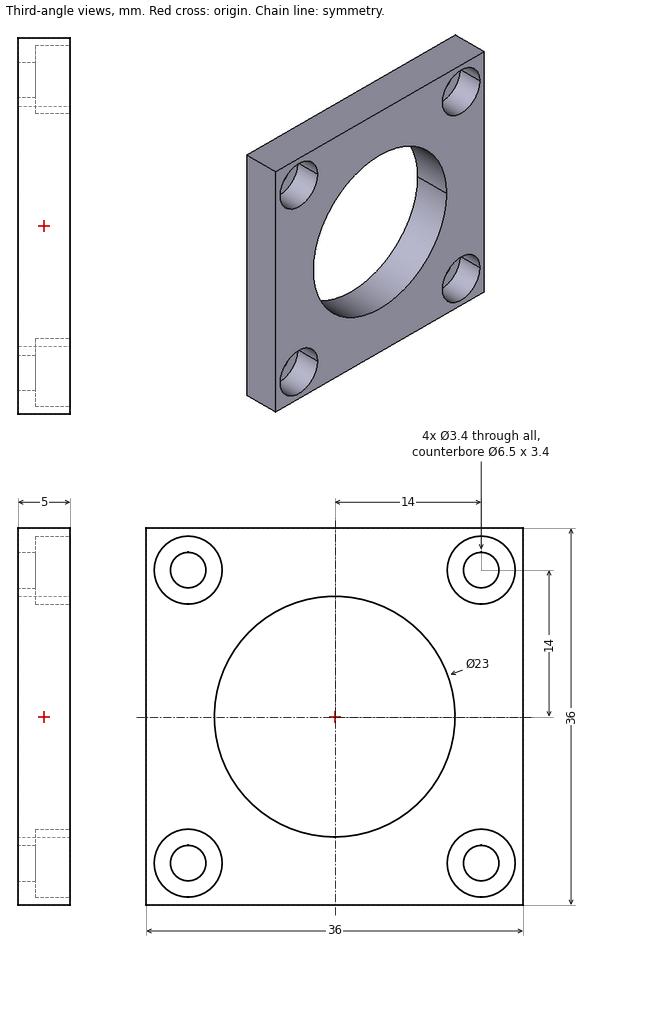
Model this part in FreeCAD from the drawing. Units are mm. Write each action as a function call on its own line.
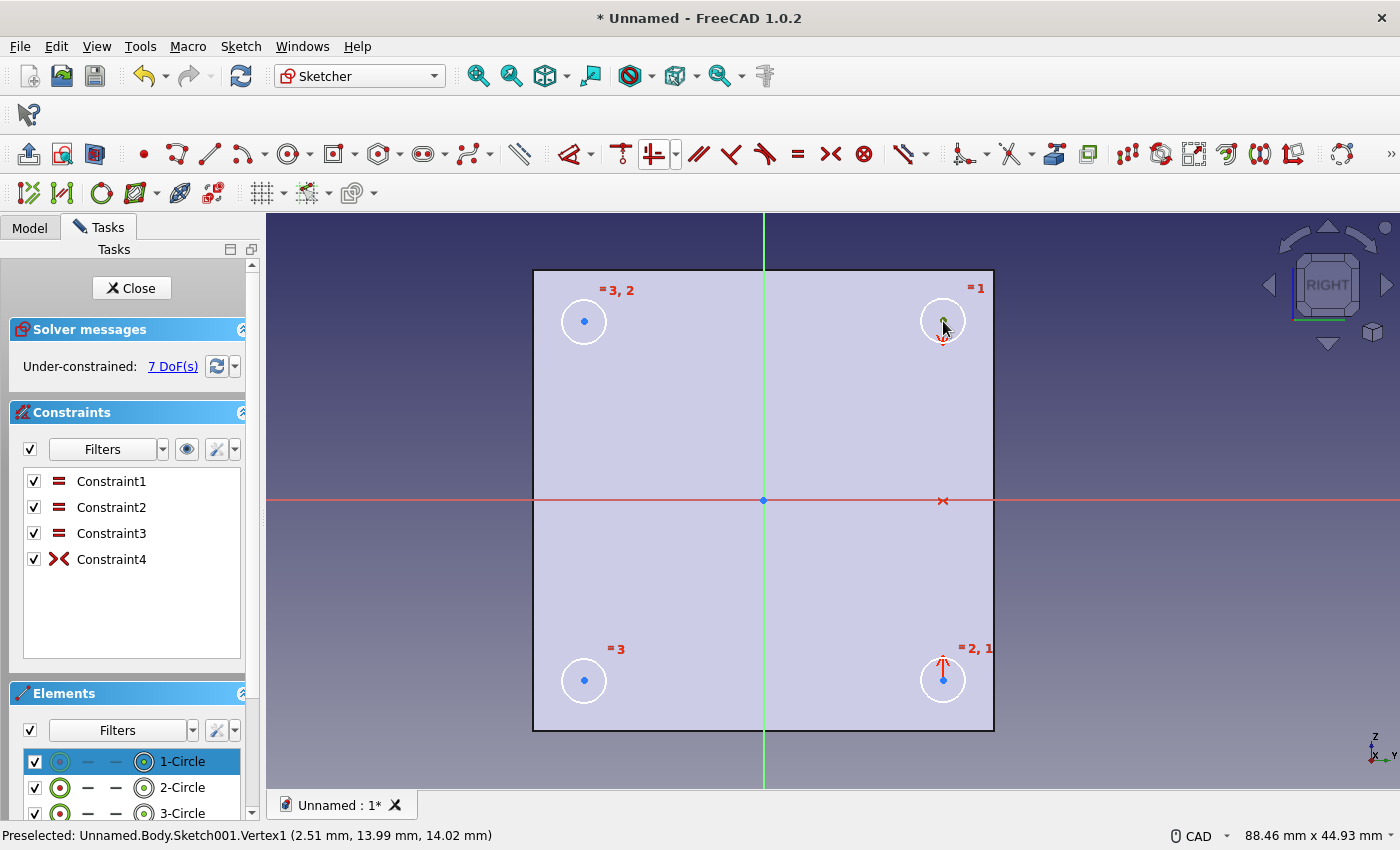
click(584, 322)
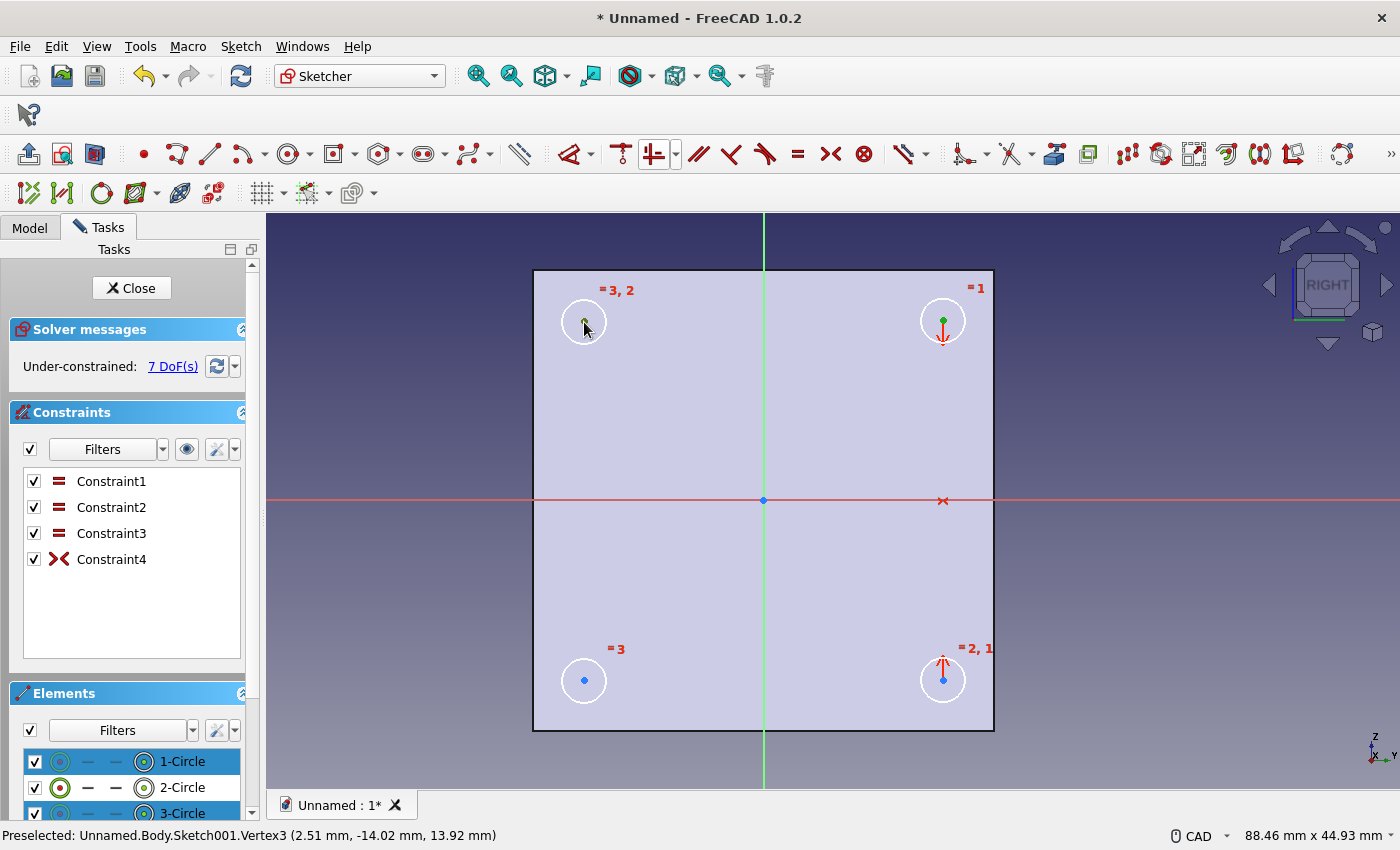
click(764, 724)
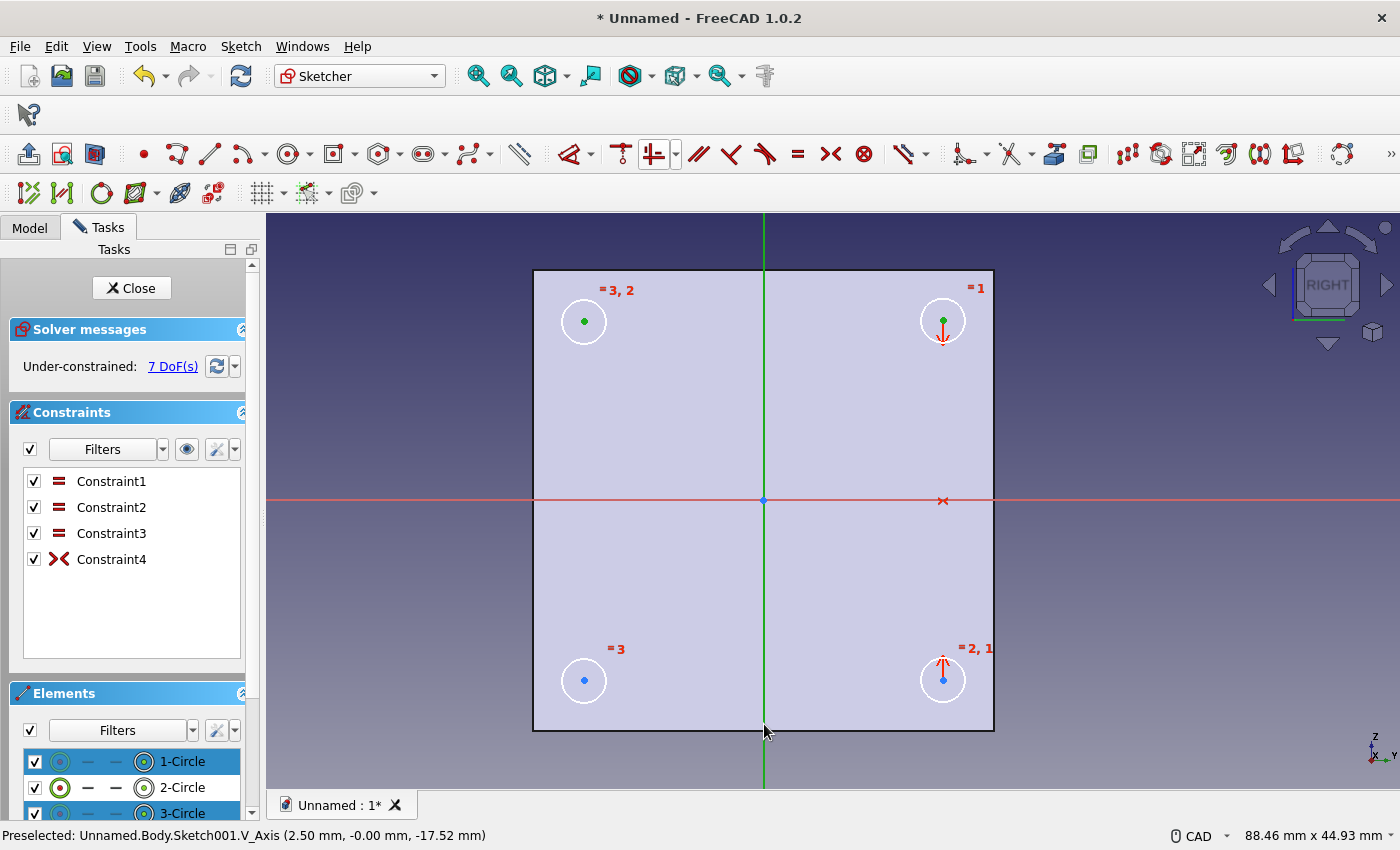
click(831, 154)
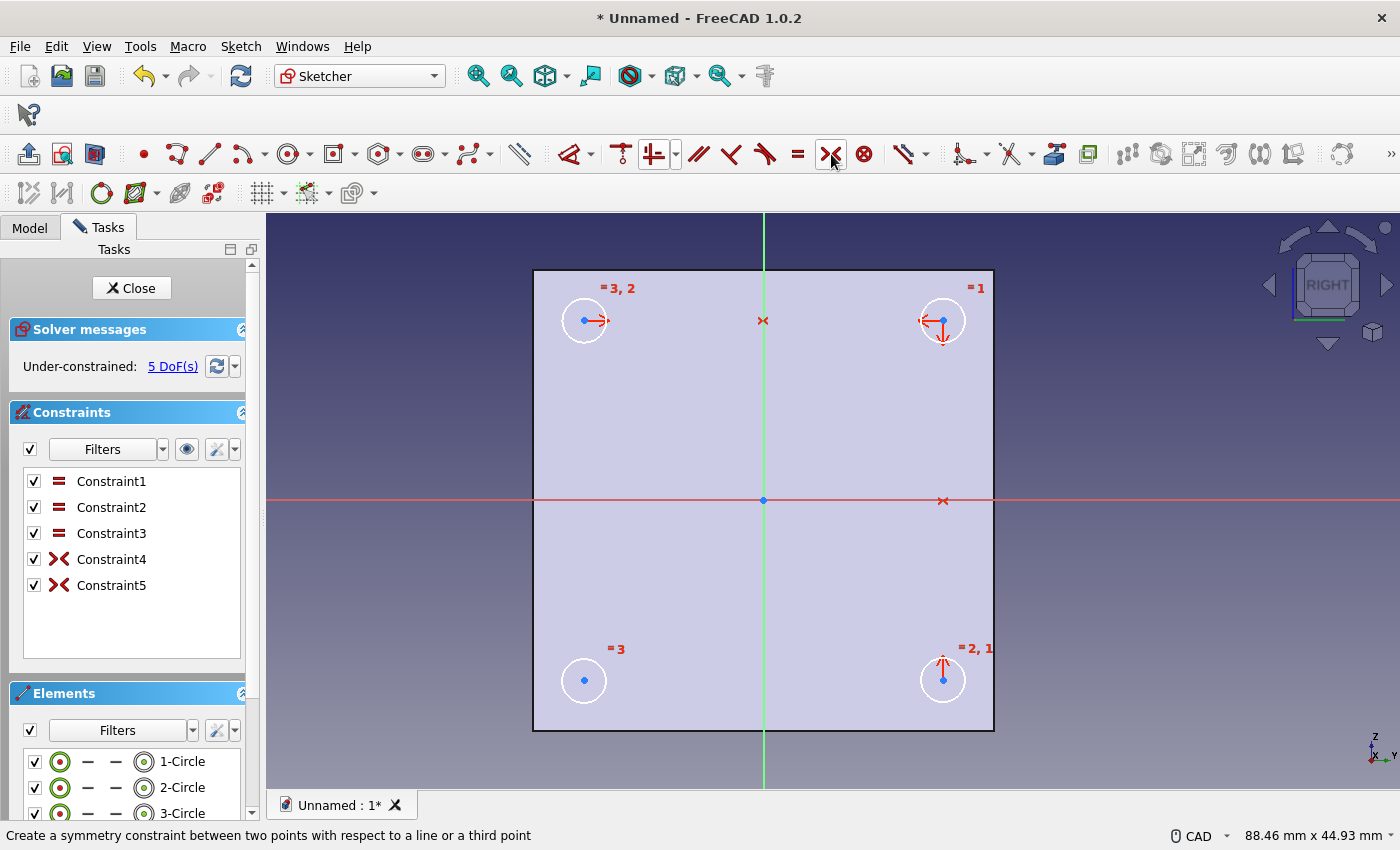
click(943, 680)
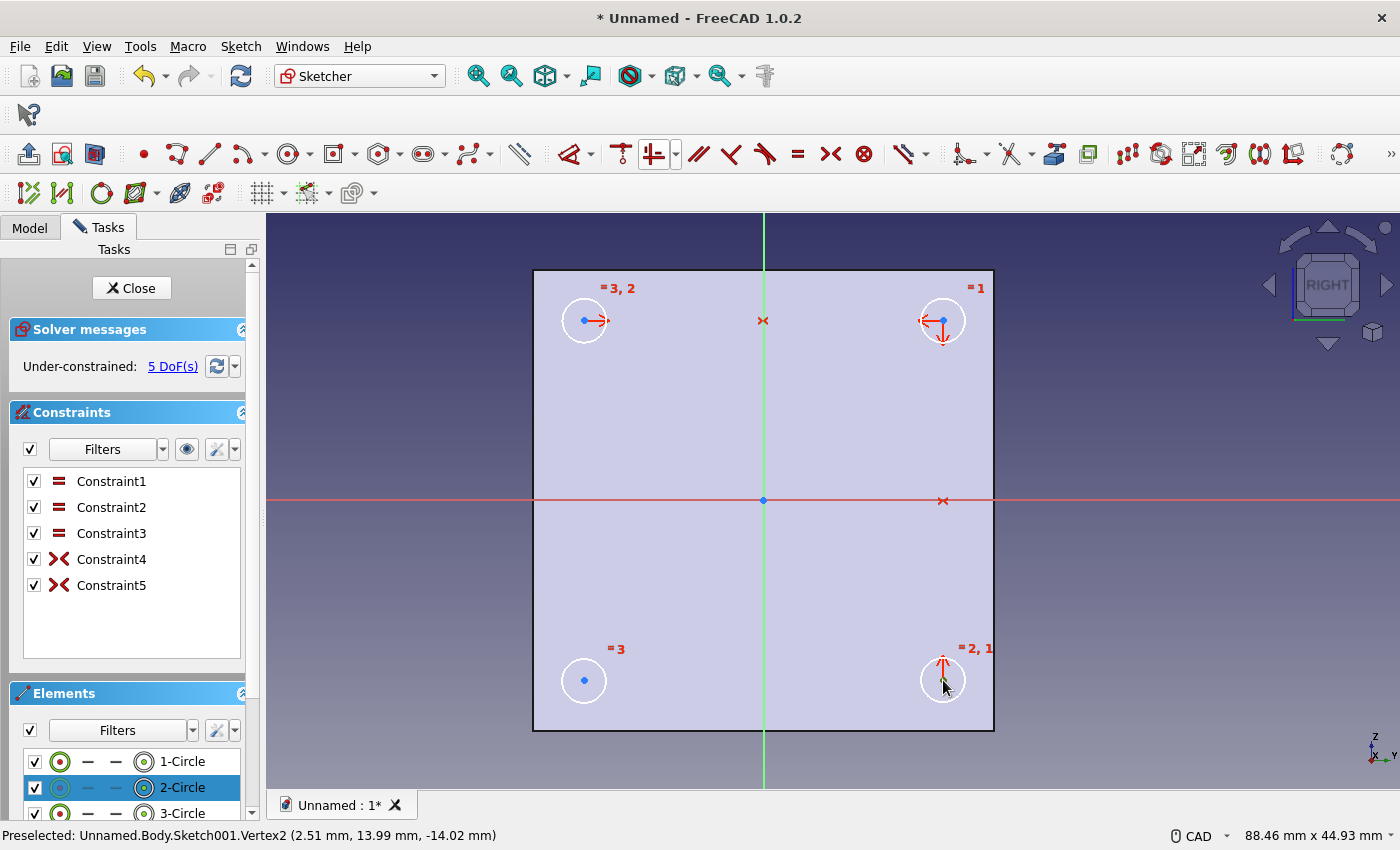
click(584, 681)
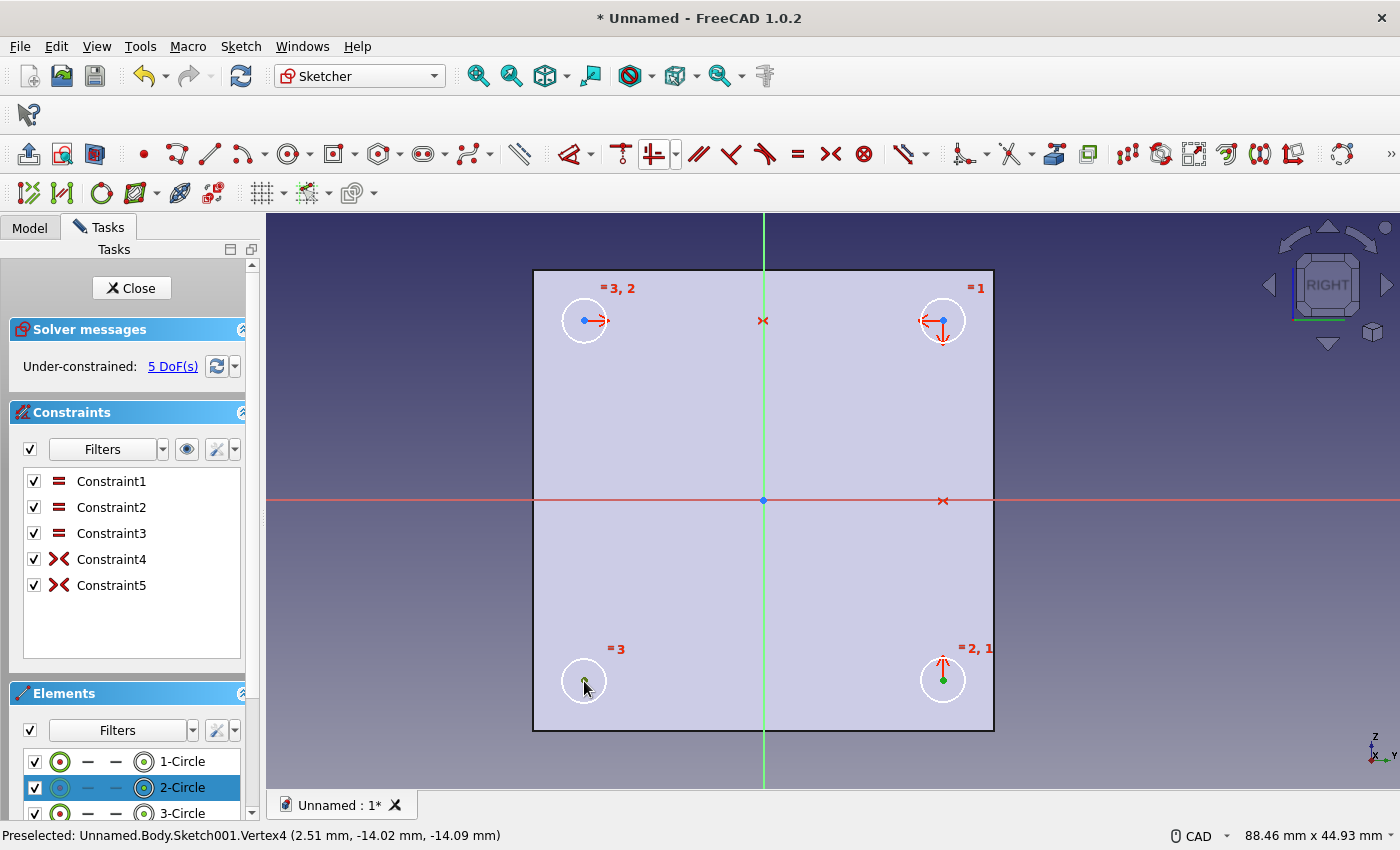
click(764, 724)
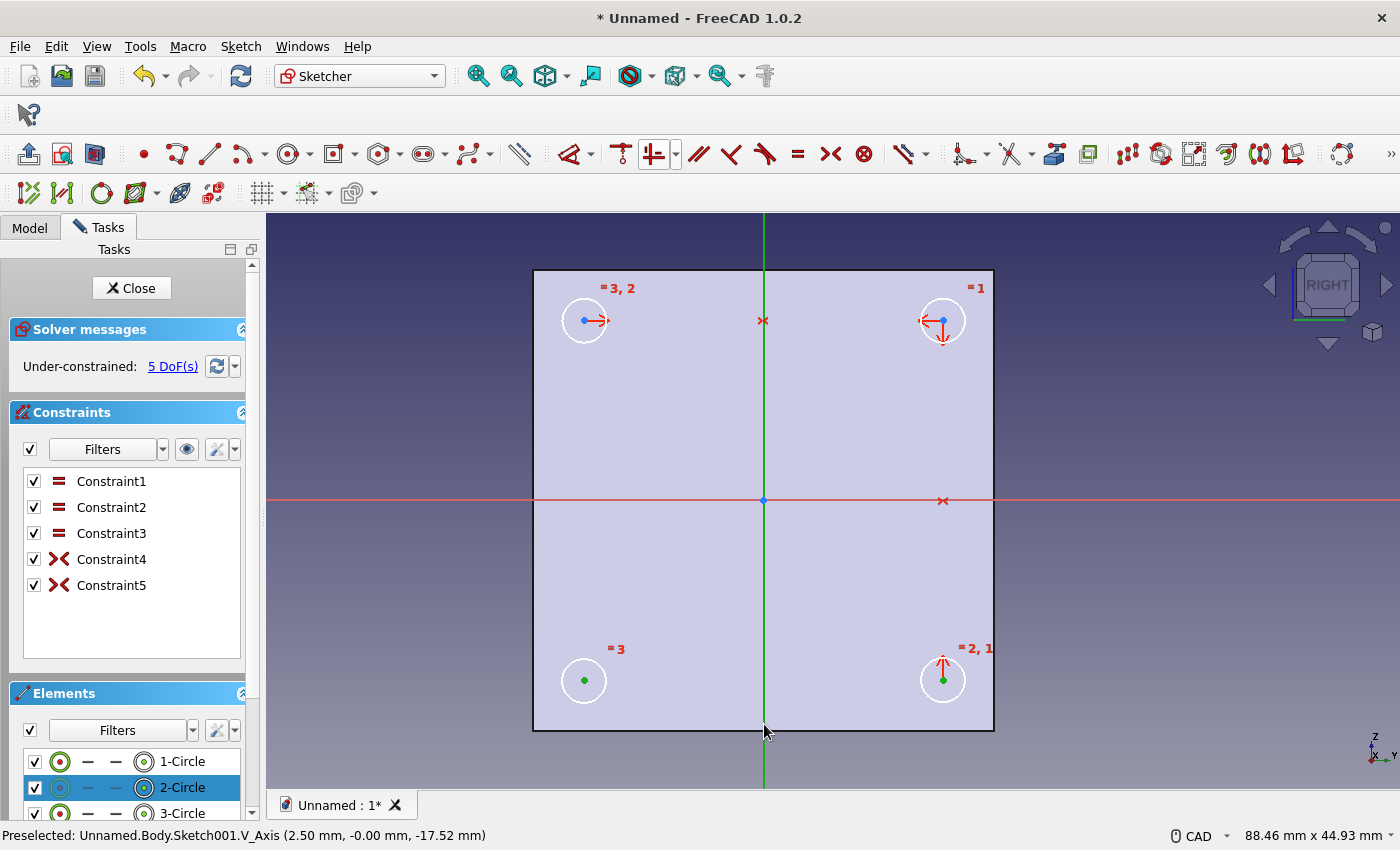
click(831, 154)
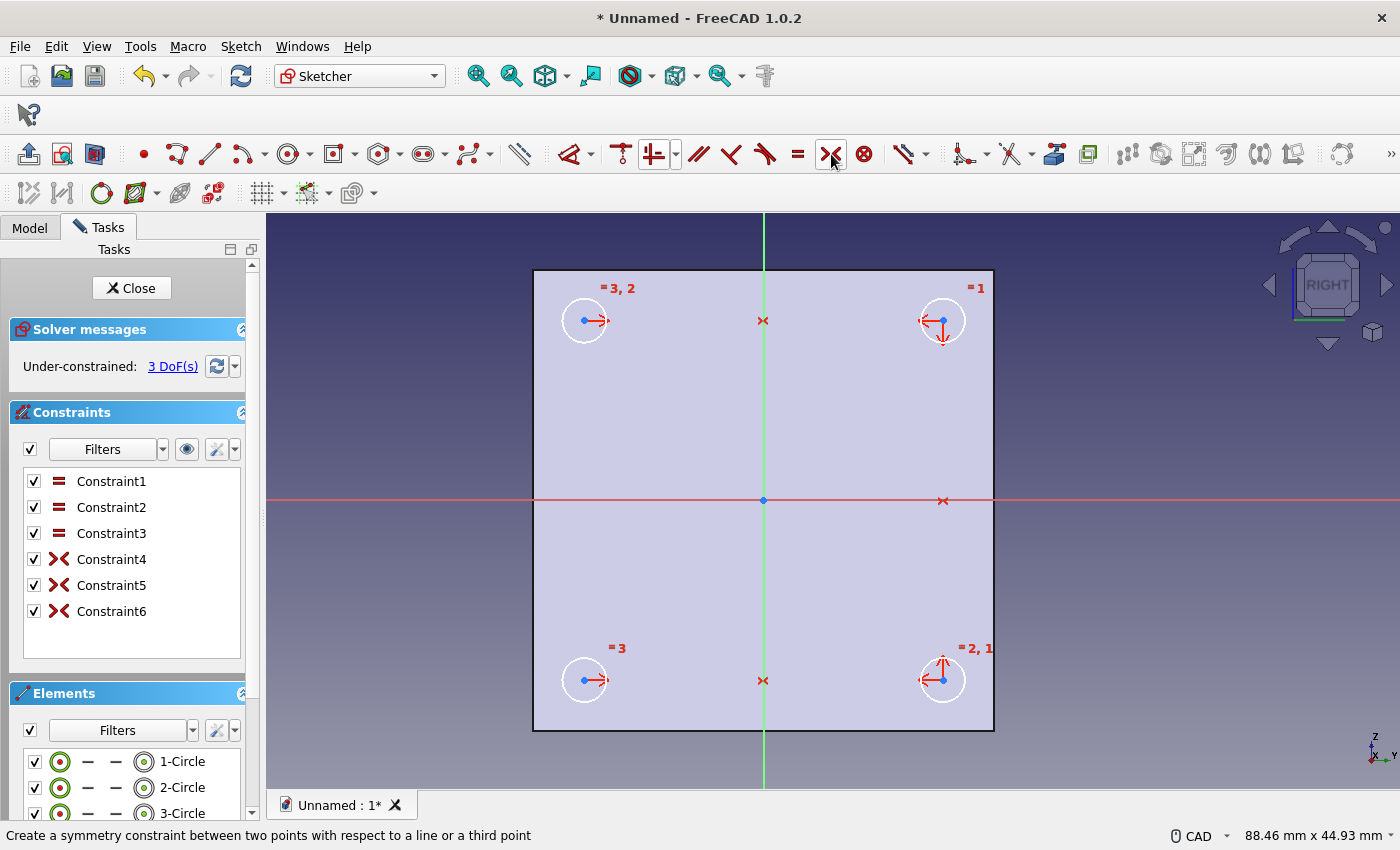
click(958, 305)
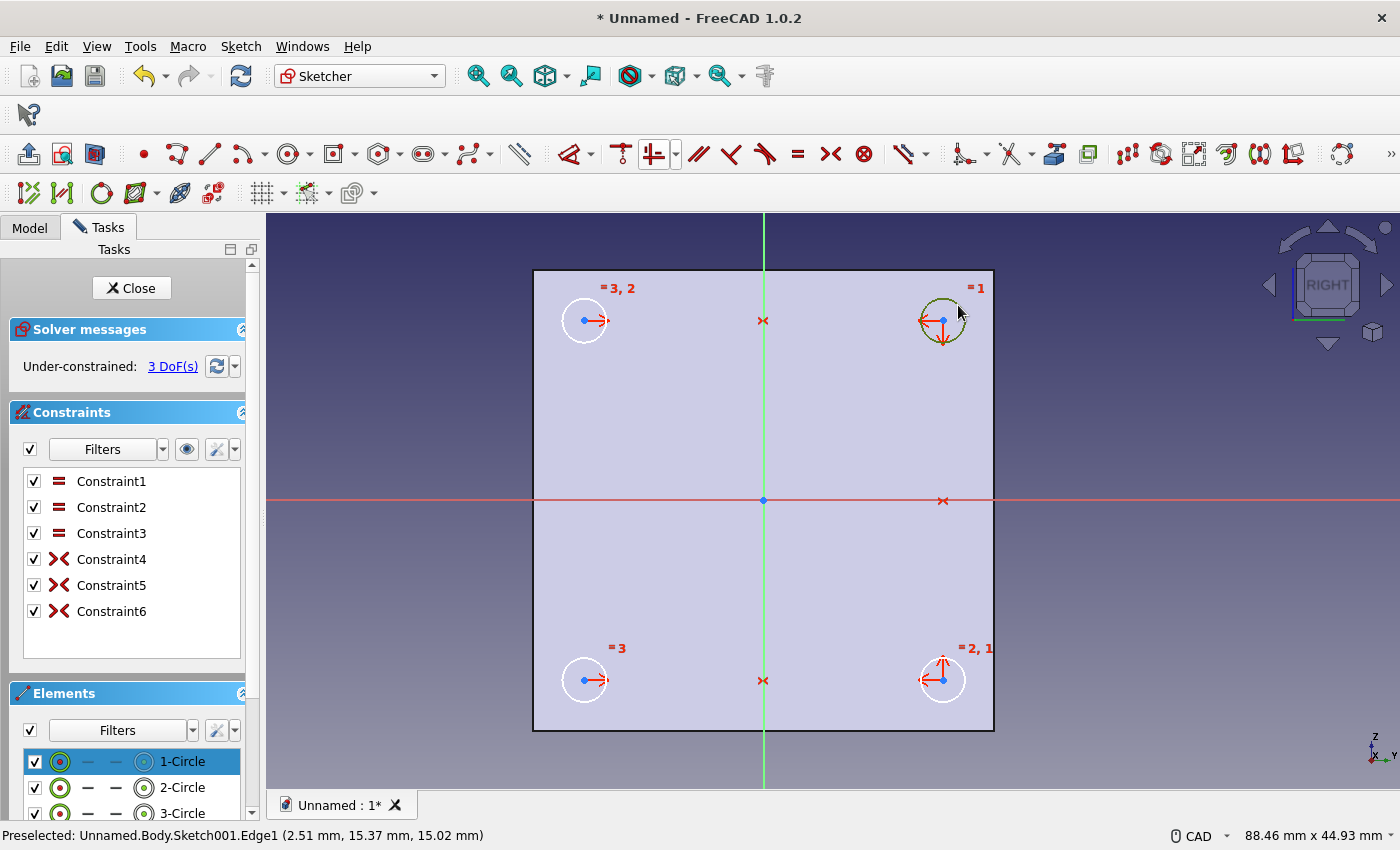
click(590, 154)